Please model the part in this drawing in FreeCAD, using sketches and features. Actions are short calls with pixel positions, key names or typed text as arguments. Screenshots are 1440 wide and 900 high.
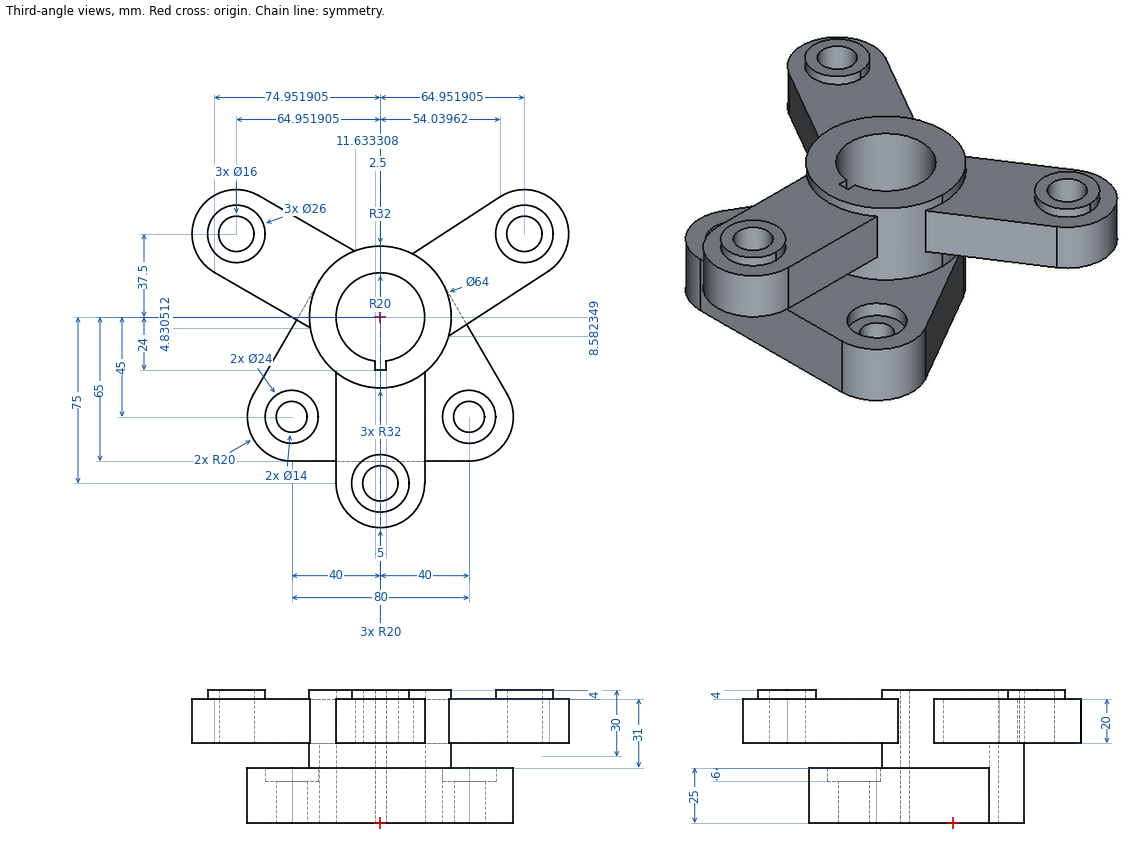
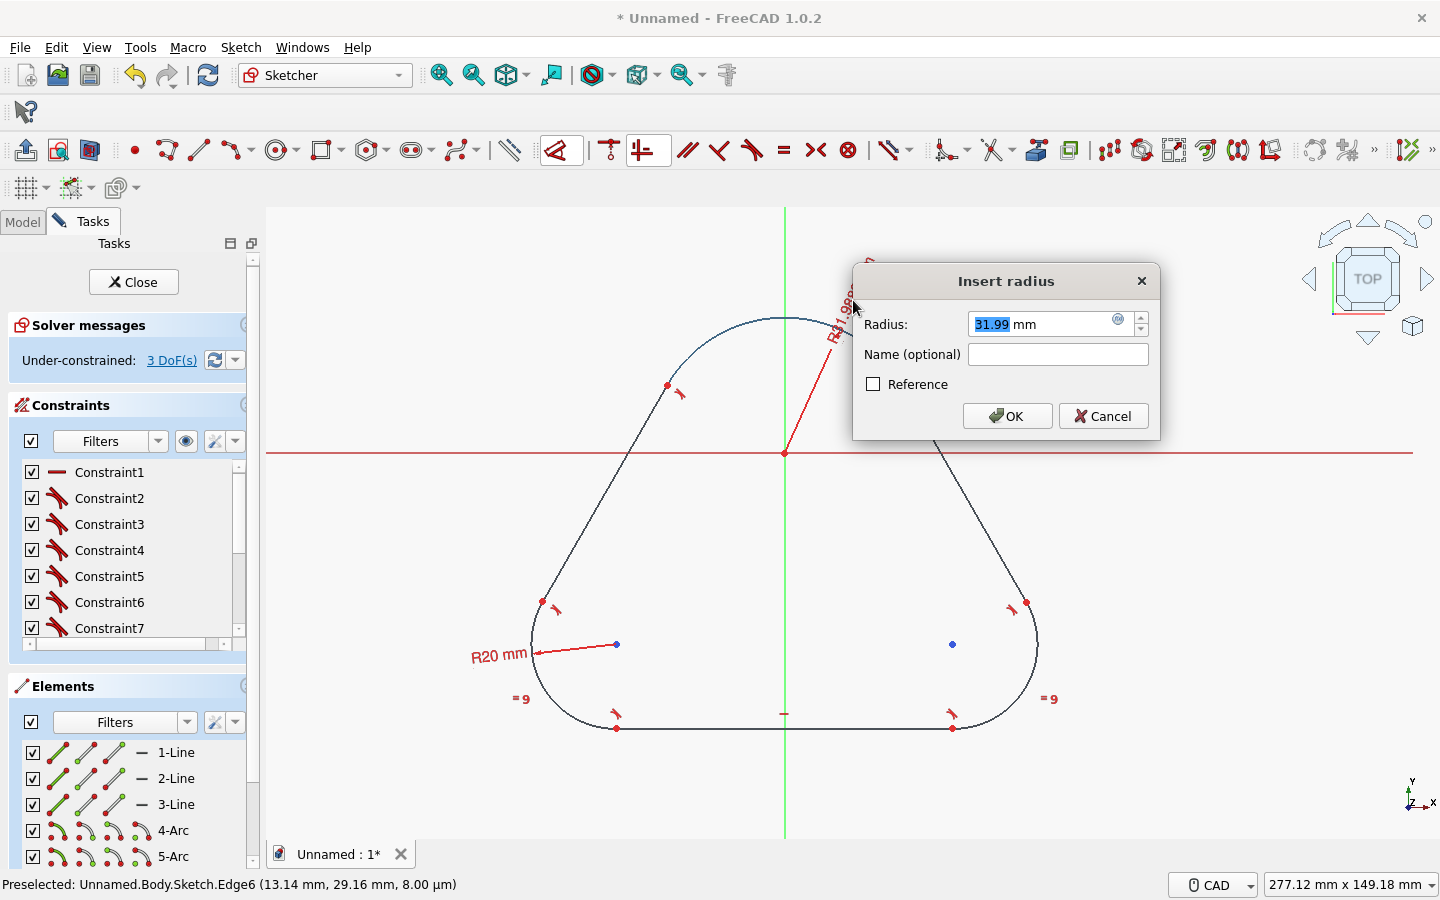
text(32)
key(Return)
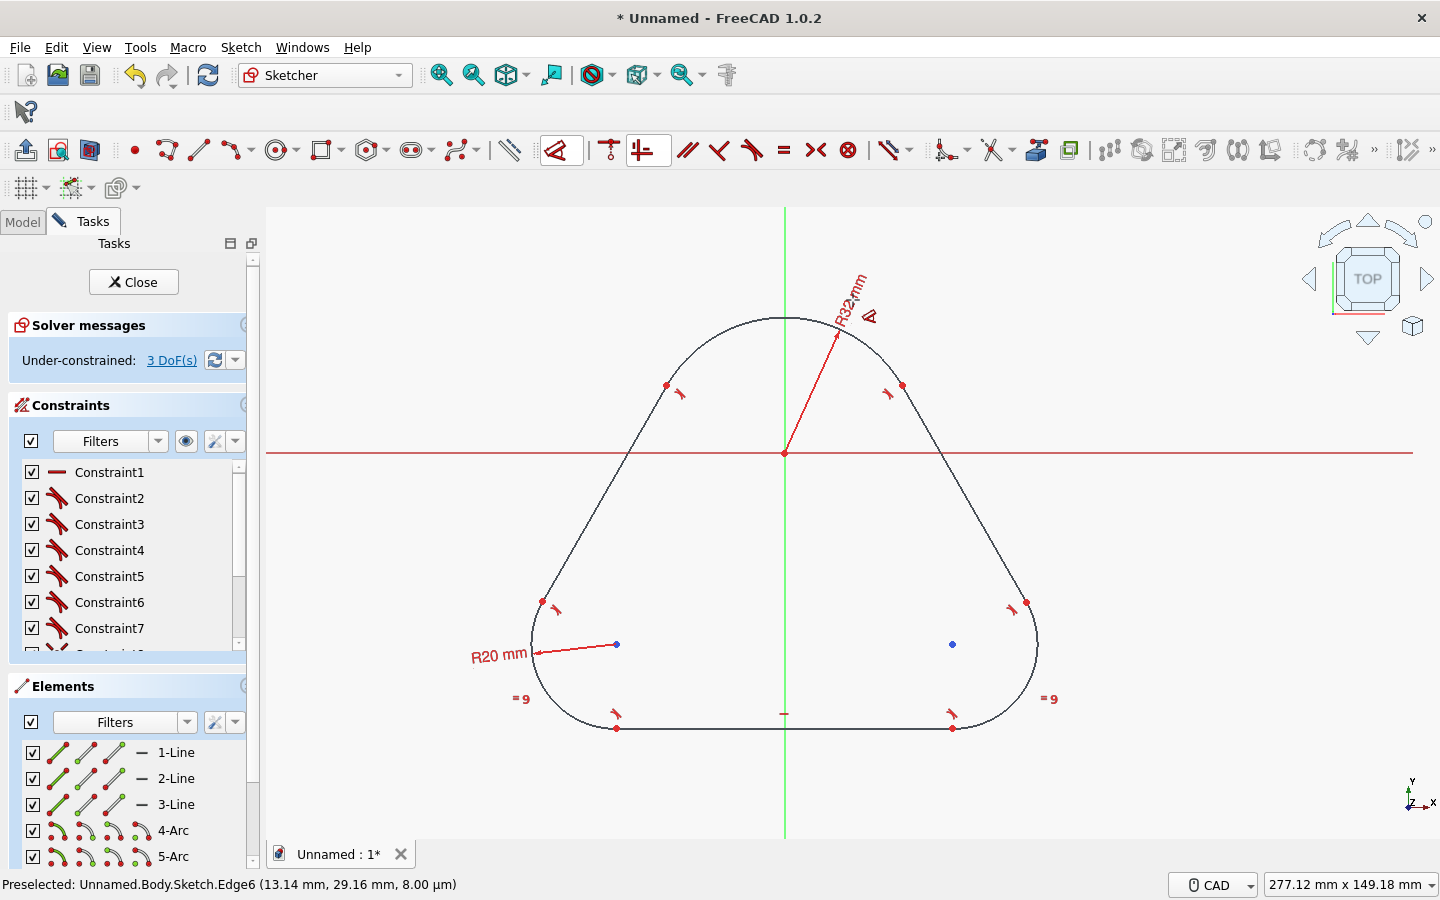
click(717, 729)
click(707, 763)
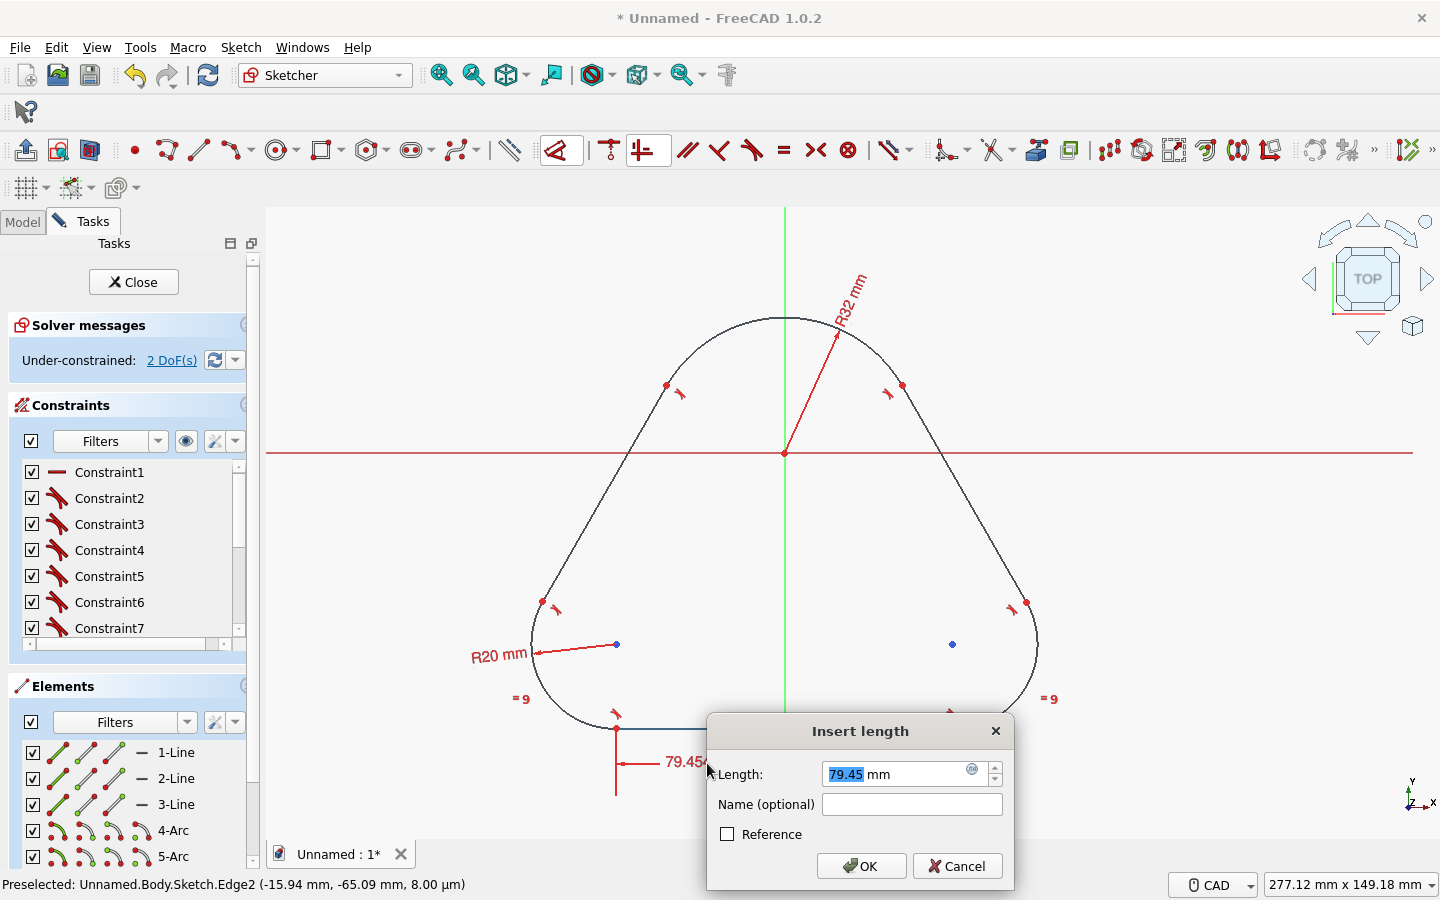
text(80)
key(Return)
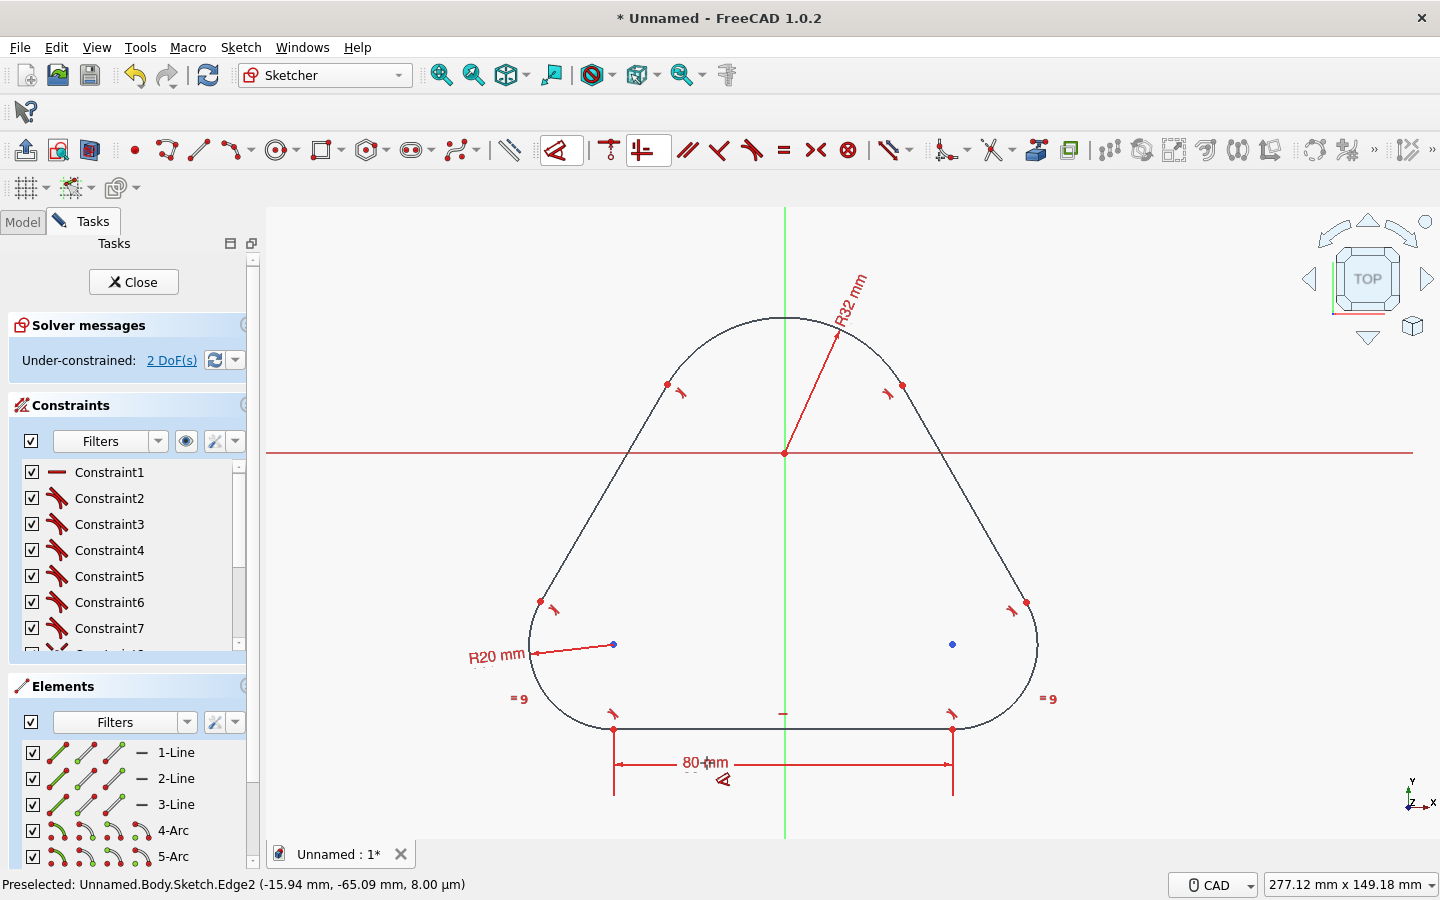
click(614, 729)
click(699, 419)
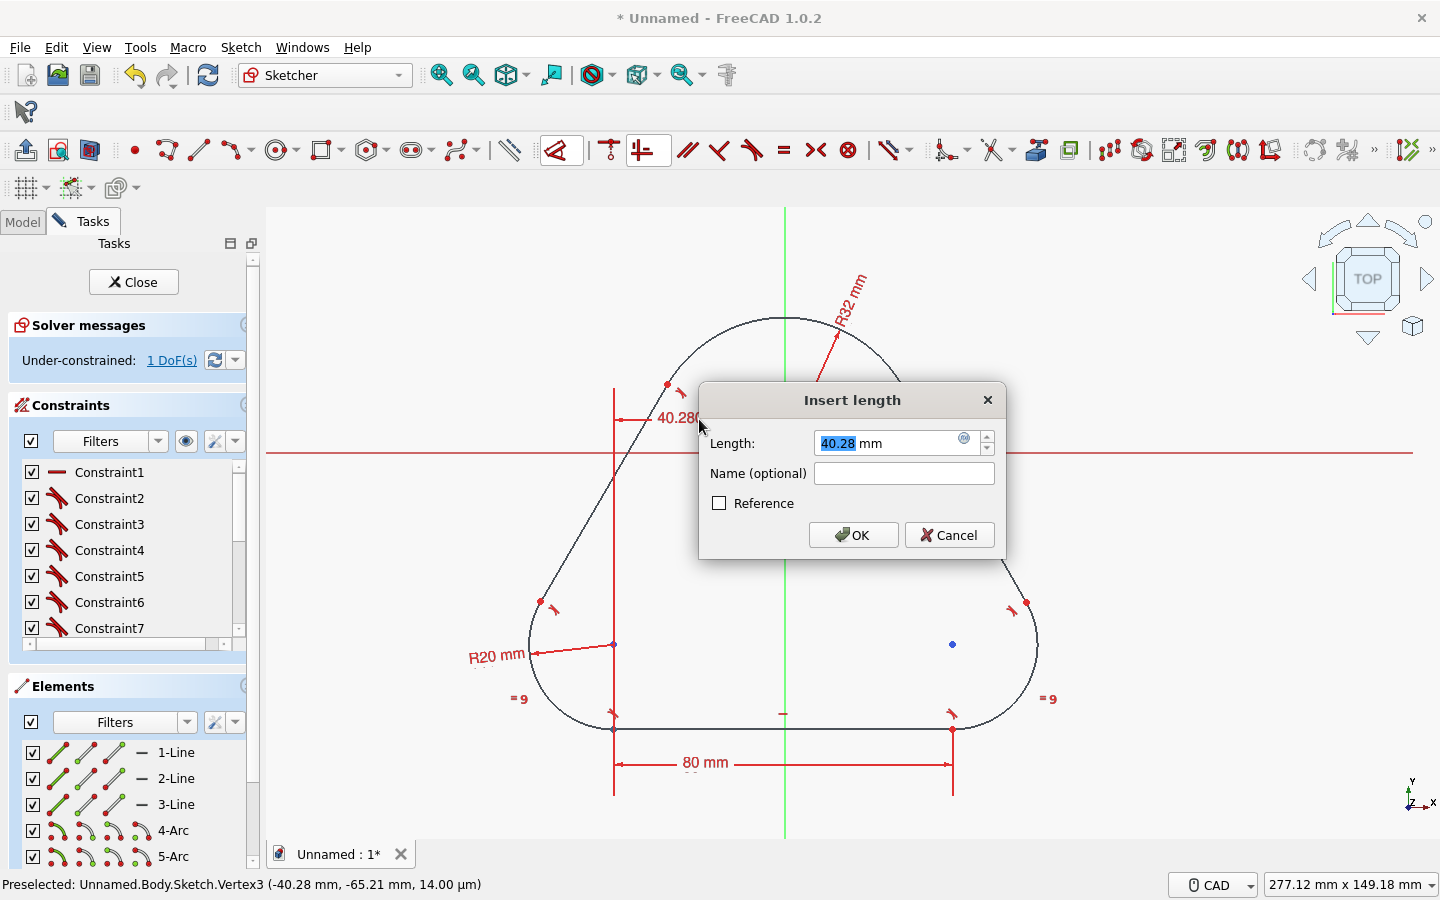
text(40)
key(Return)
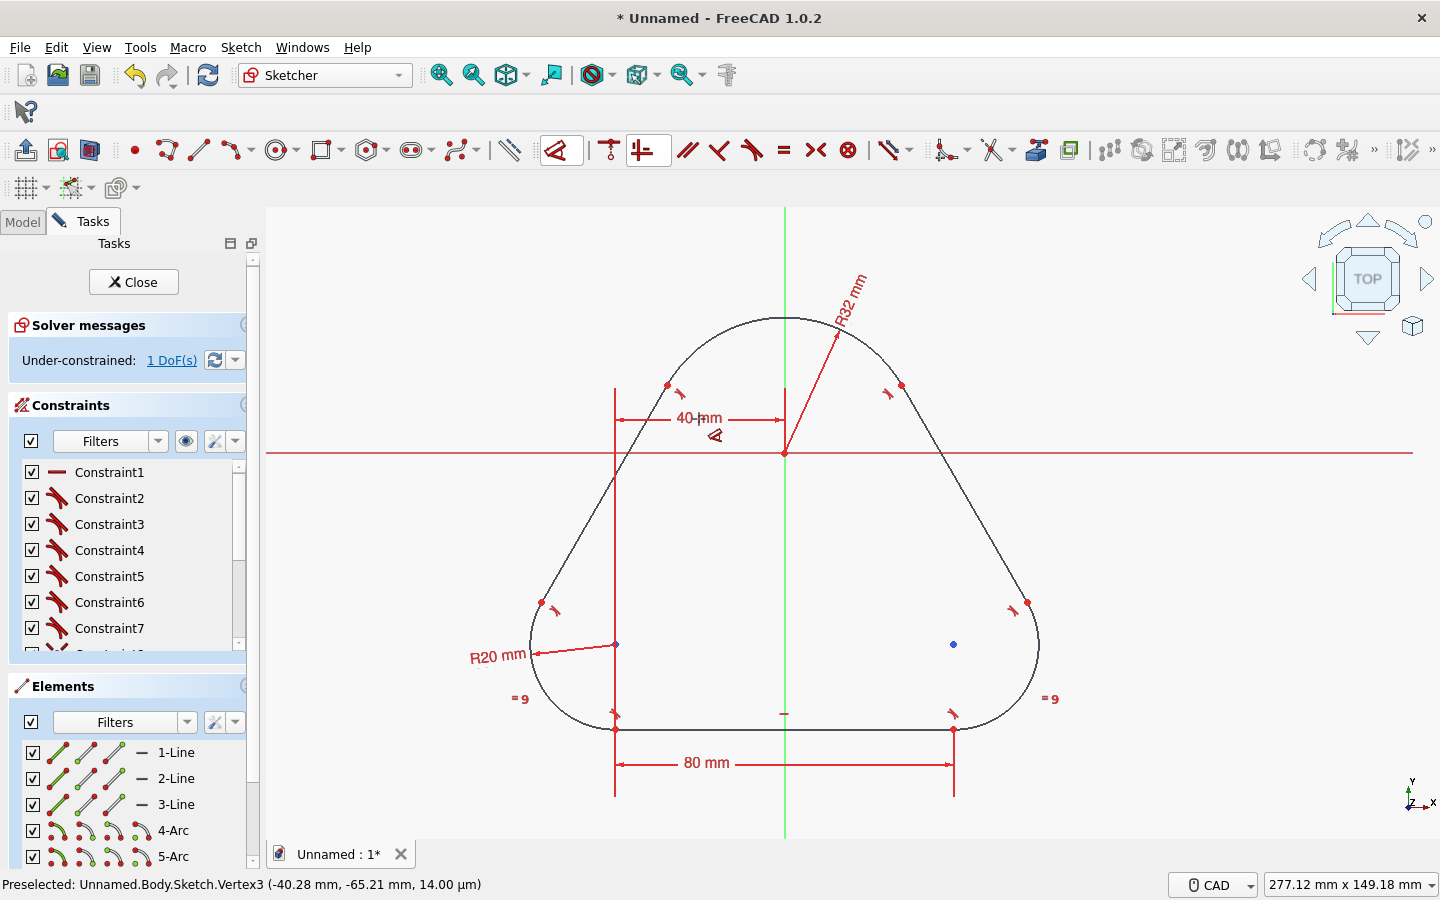
click(615, 730)
click(581, 591)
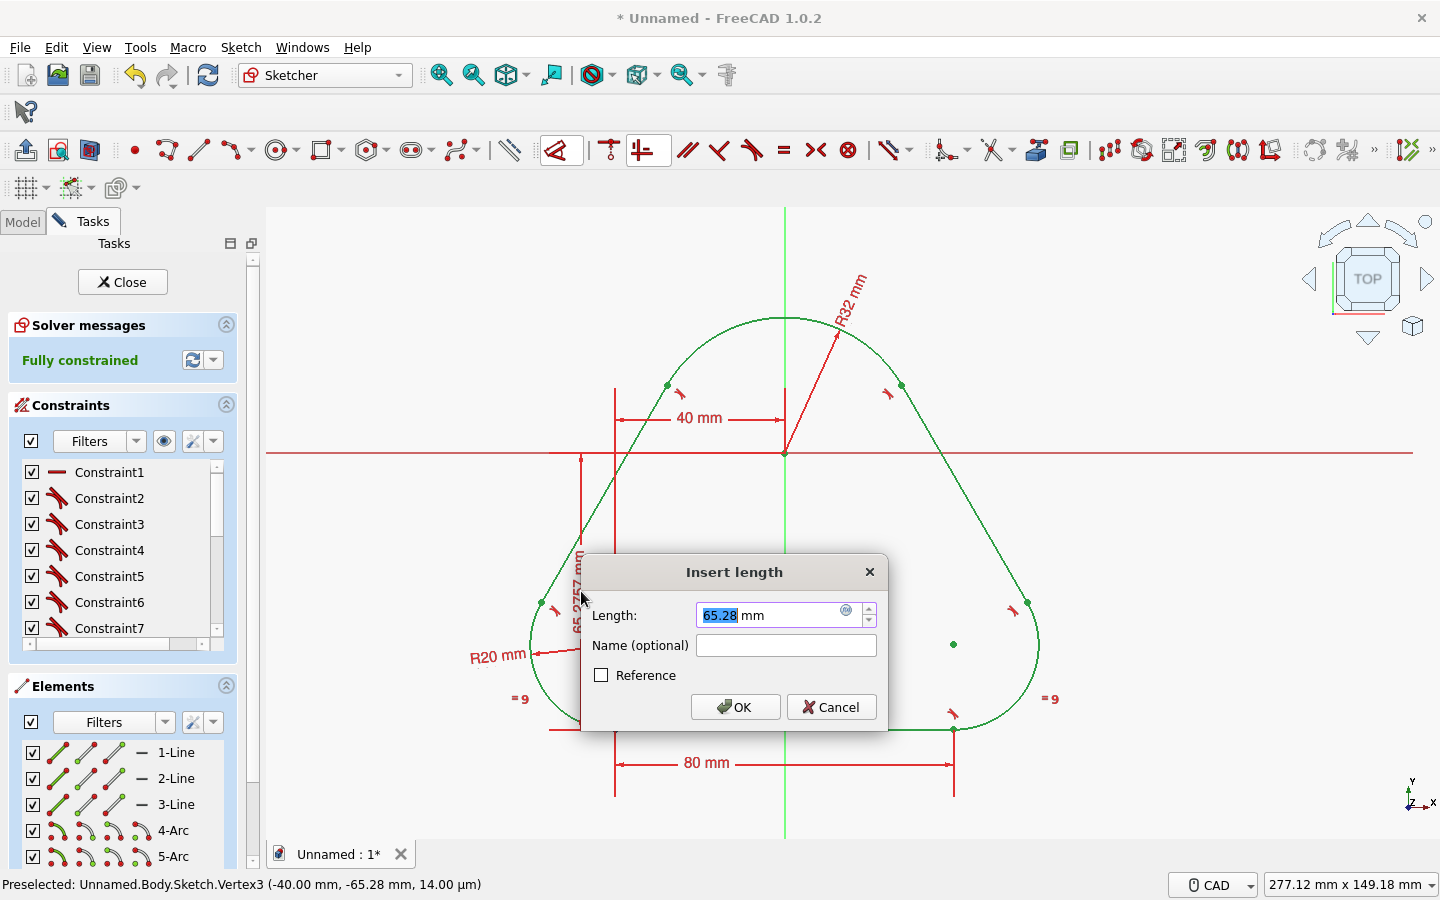
text(65)
key(Return)
key(Escape)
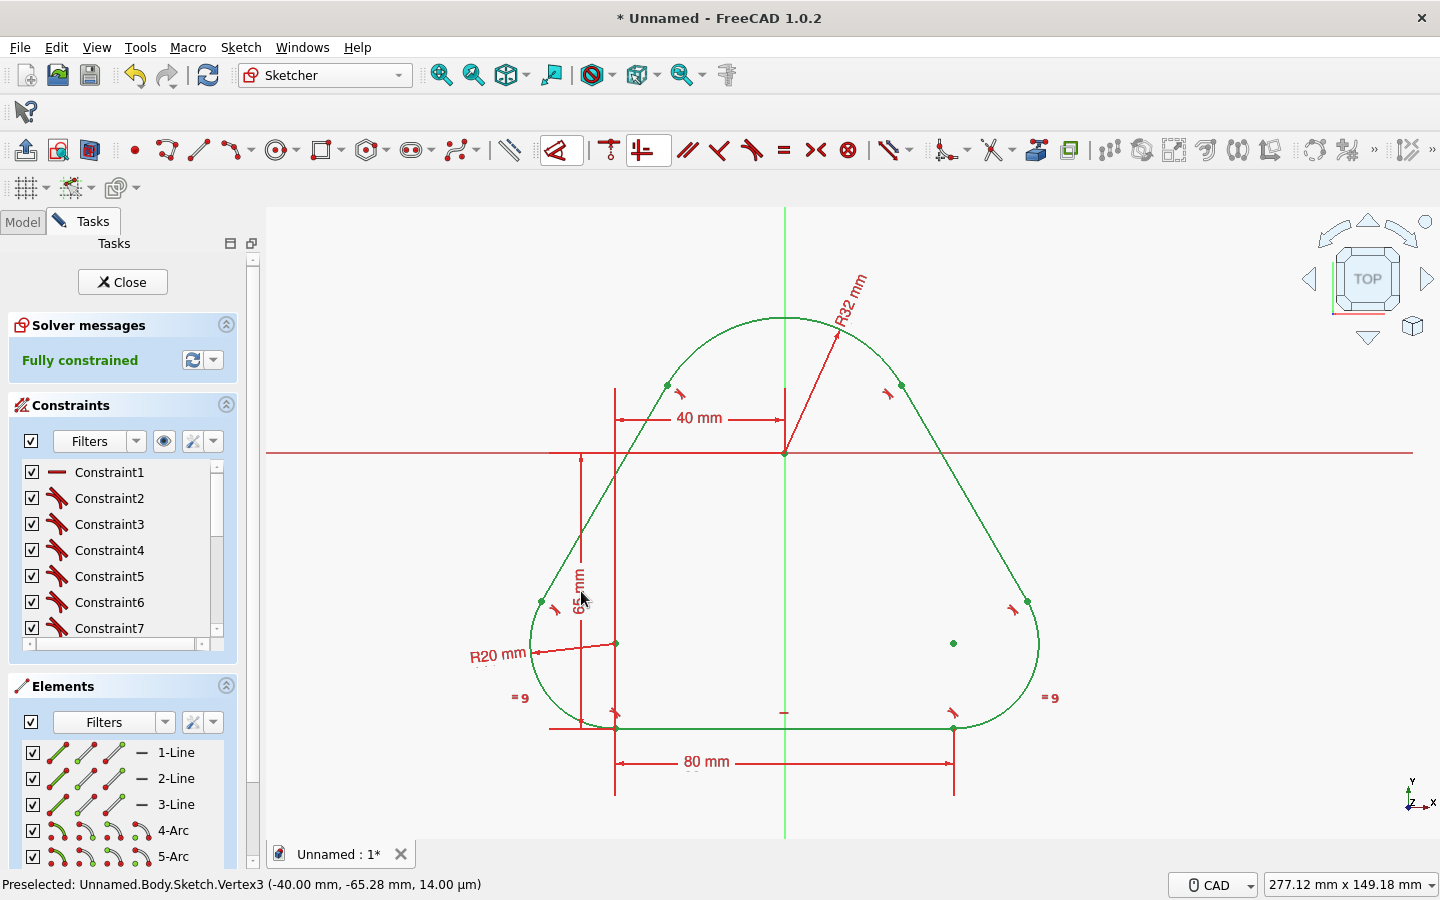
click(123, 282)